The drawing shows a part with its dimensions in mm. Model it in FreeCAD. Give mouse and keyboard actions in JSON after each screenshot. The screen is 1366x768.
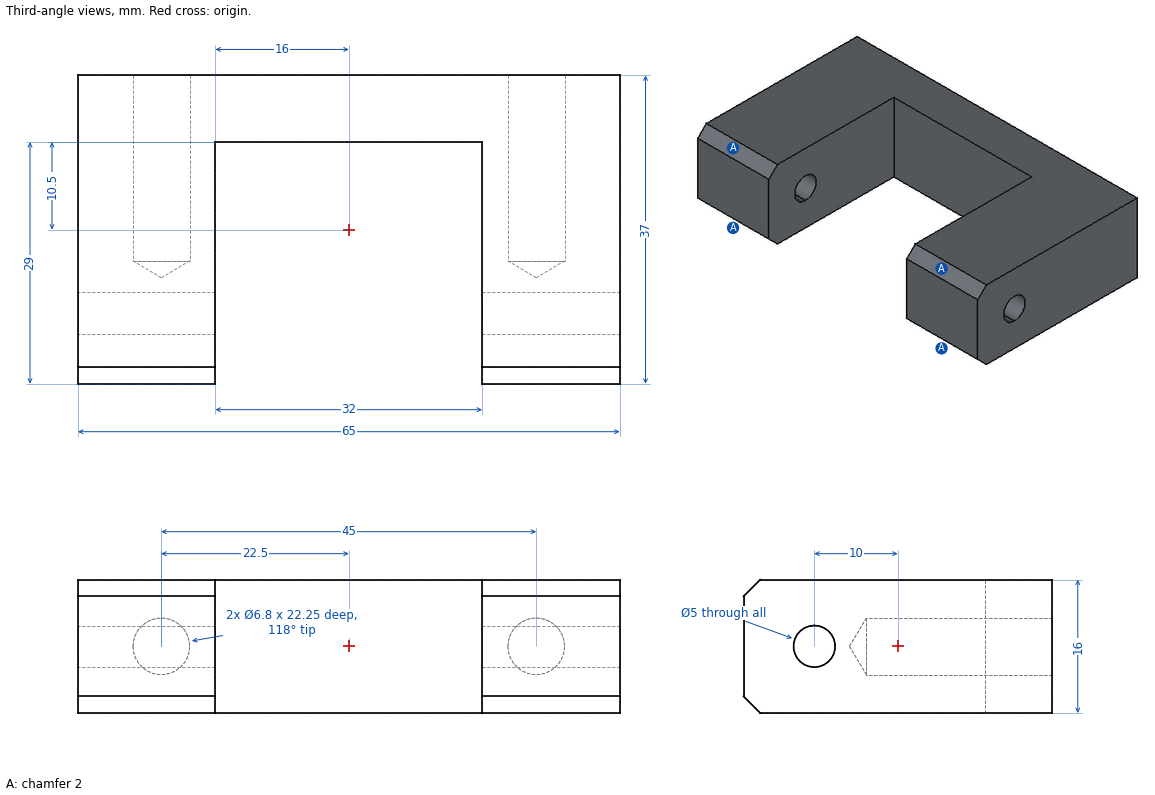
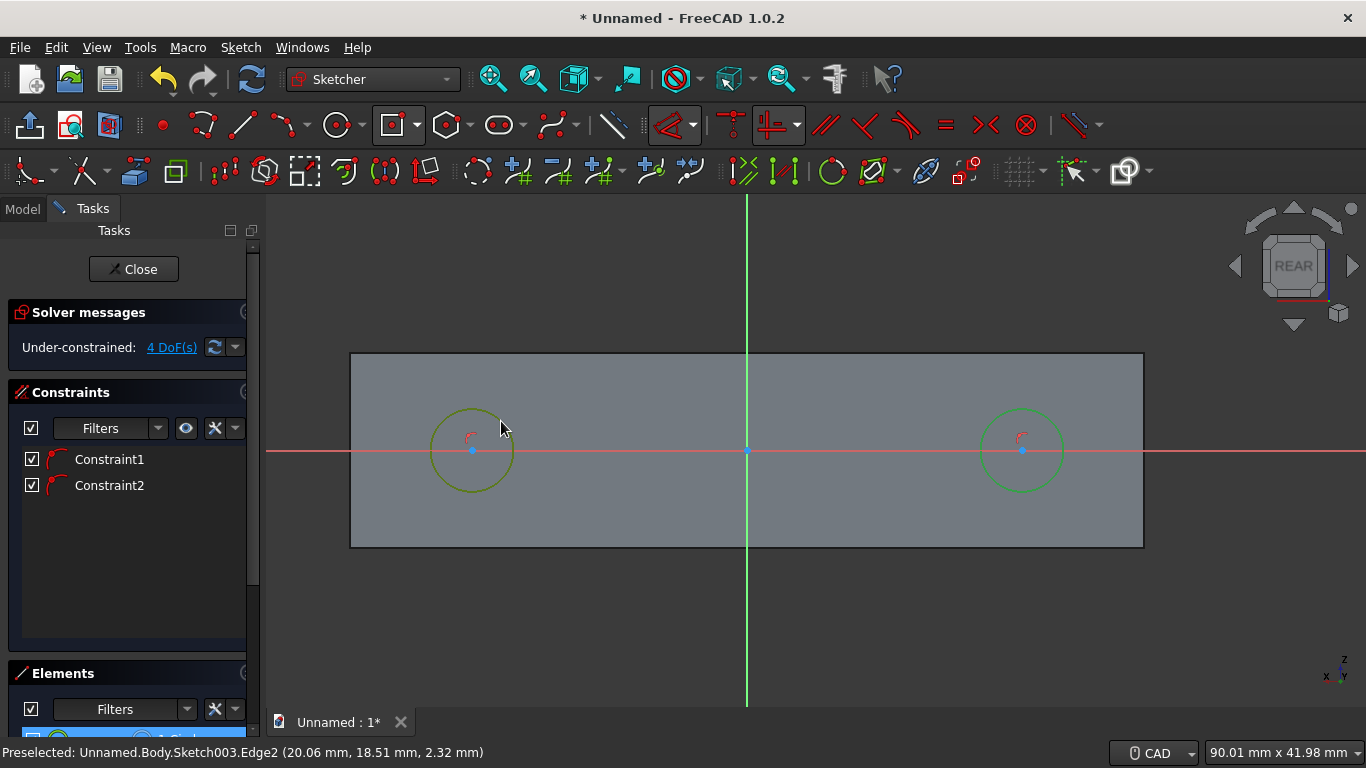
{"action": "left_click", "coordinate": [946, 126]}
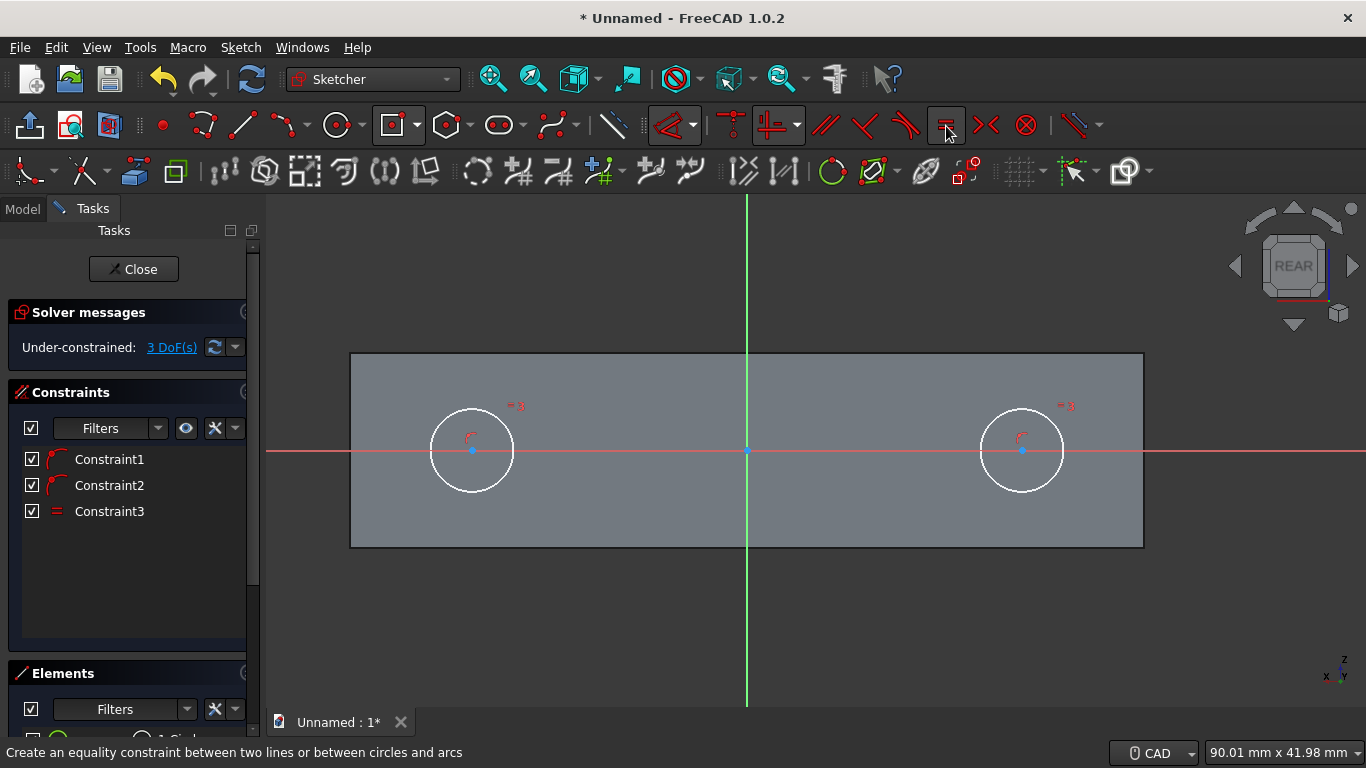
{"action": "left_click", "coordinate": [1051, 421]}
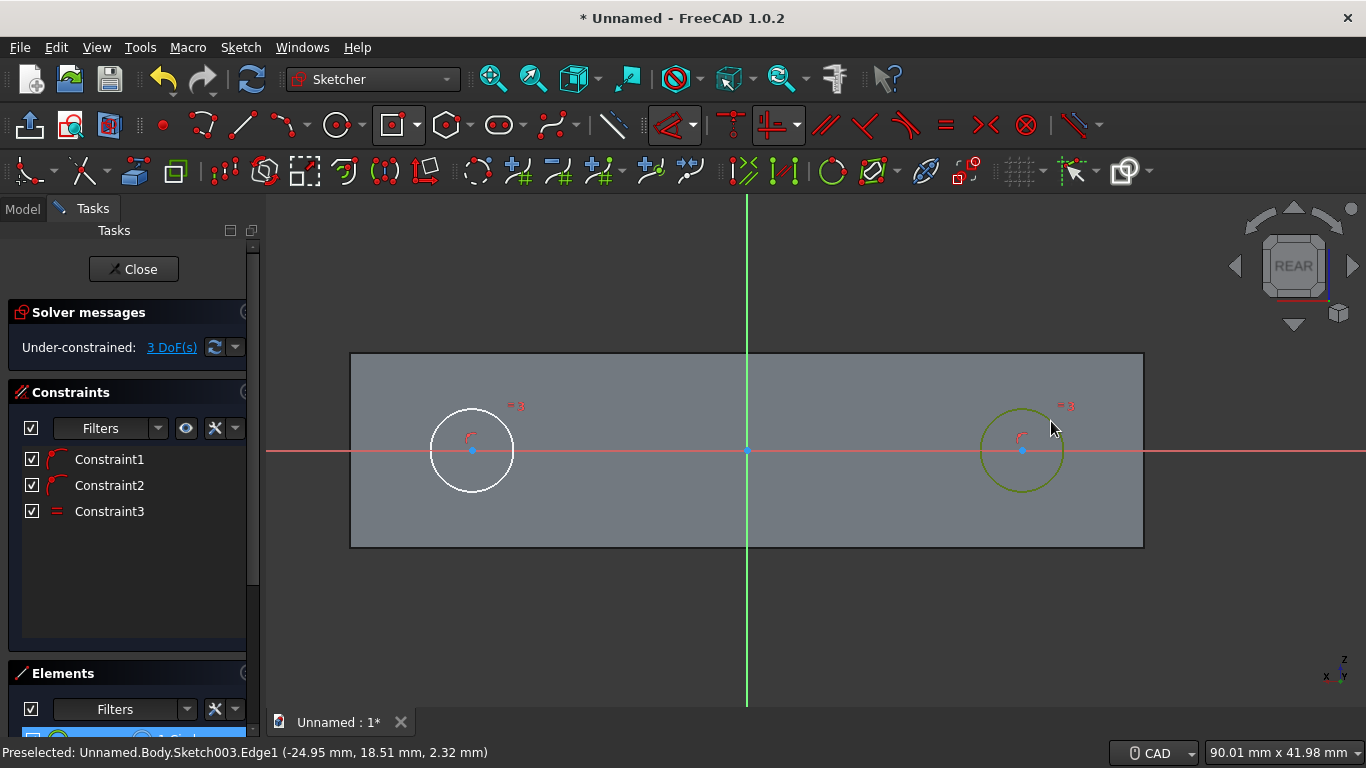
{"action": "left_click", "coordinate": [696, 126]}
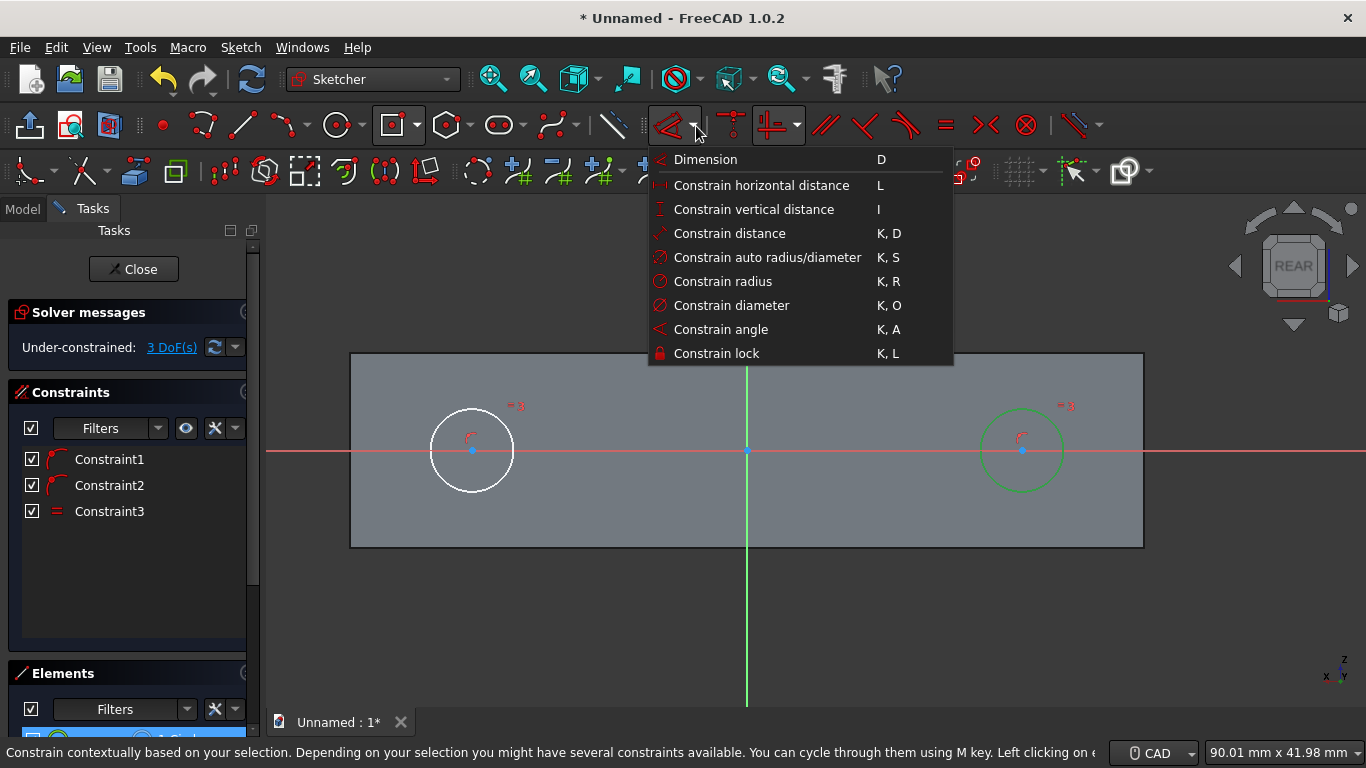
{"action": "left_click", "coordinate": [801, 305]}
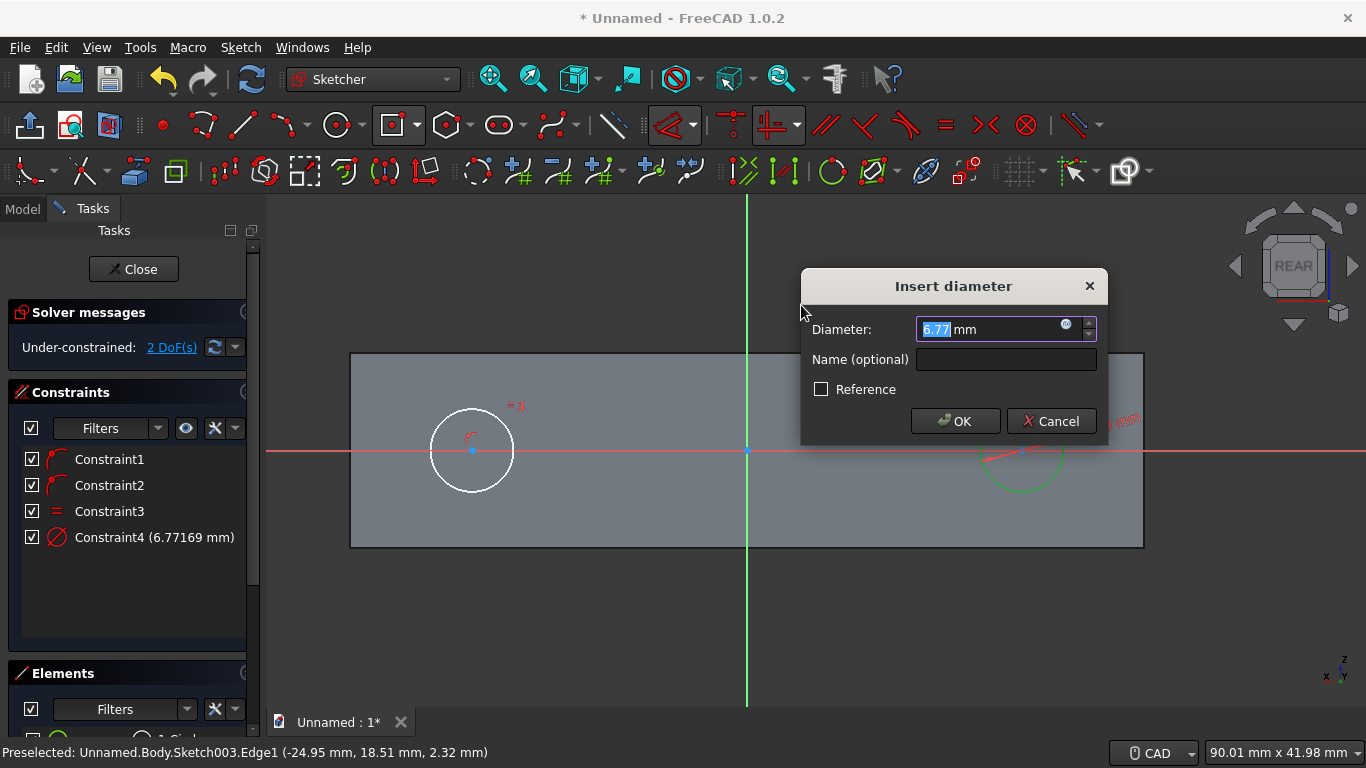
{"action": "type", "text": "6.8"}
{"action": "key", "text": "Return"}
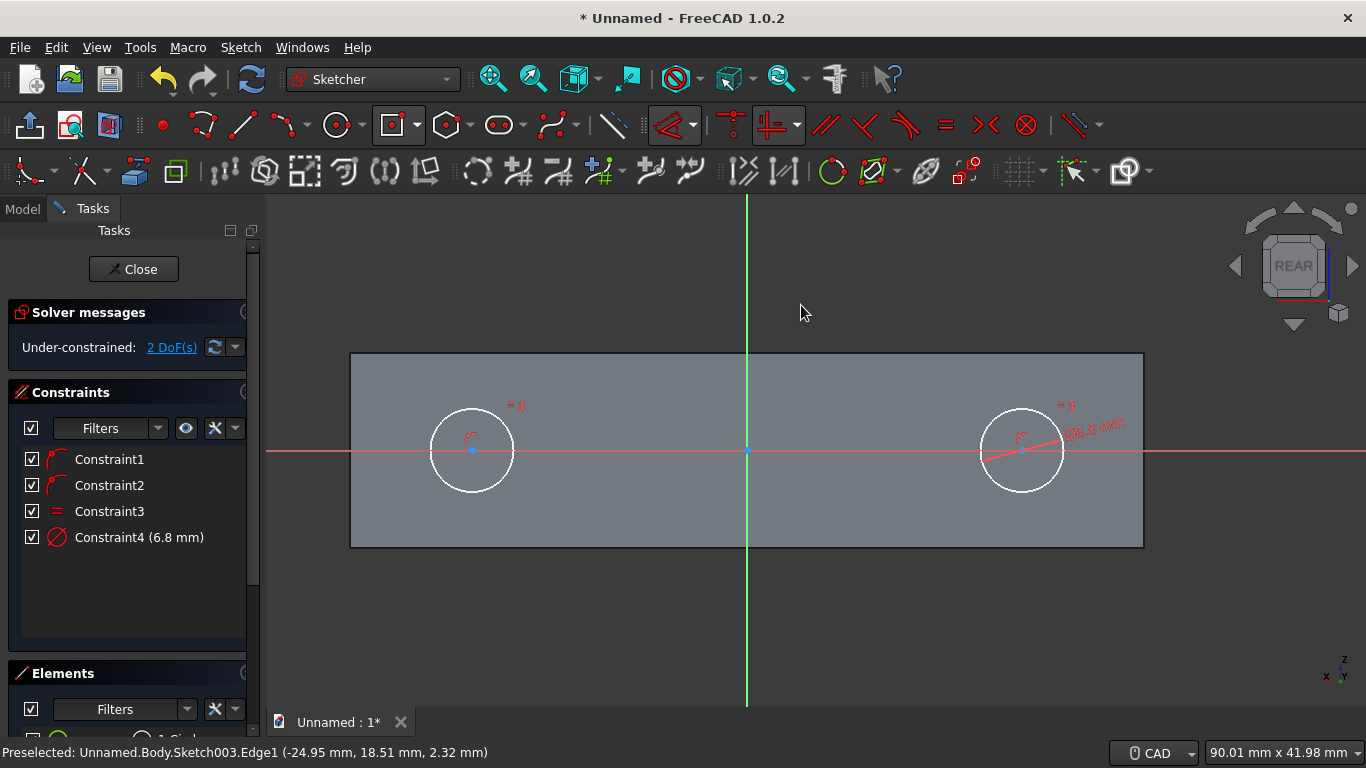
{"action": "left_click", "coordinate": [1022, 450]}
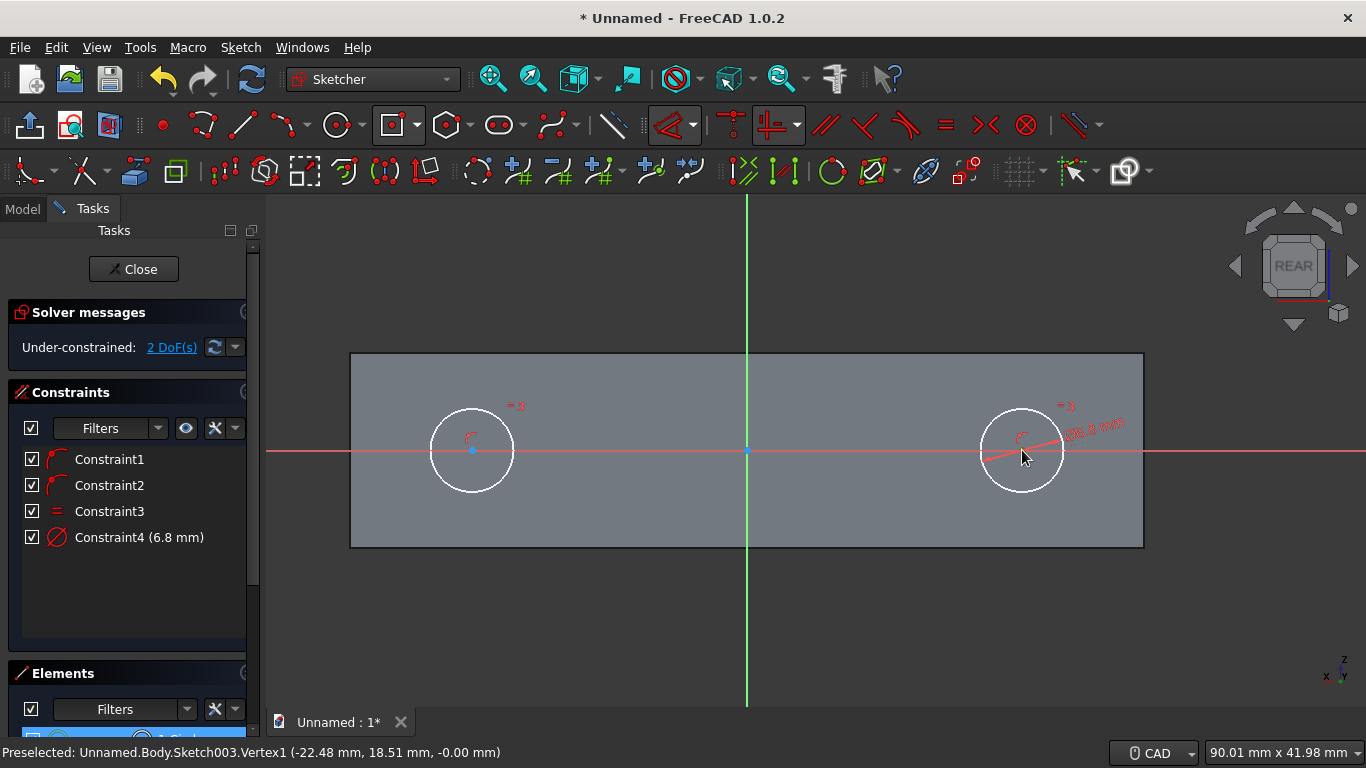
{"action": "left_click", "coordinate": [472, 450]}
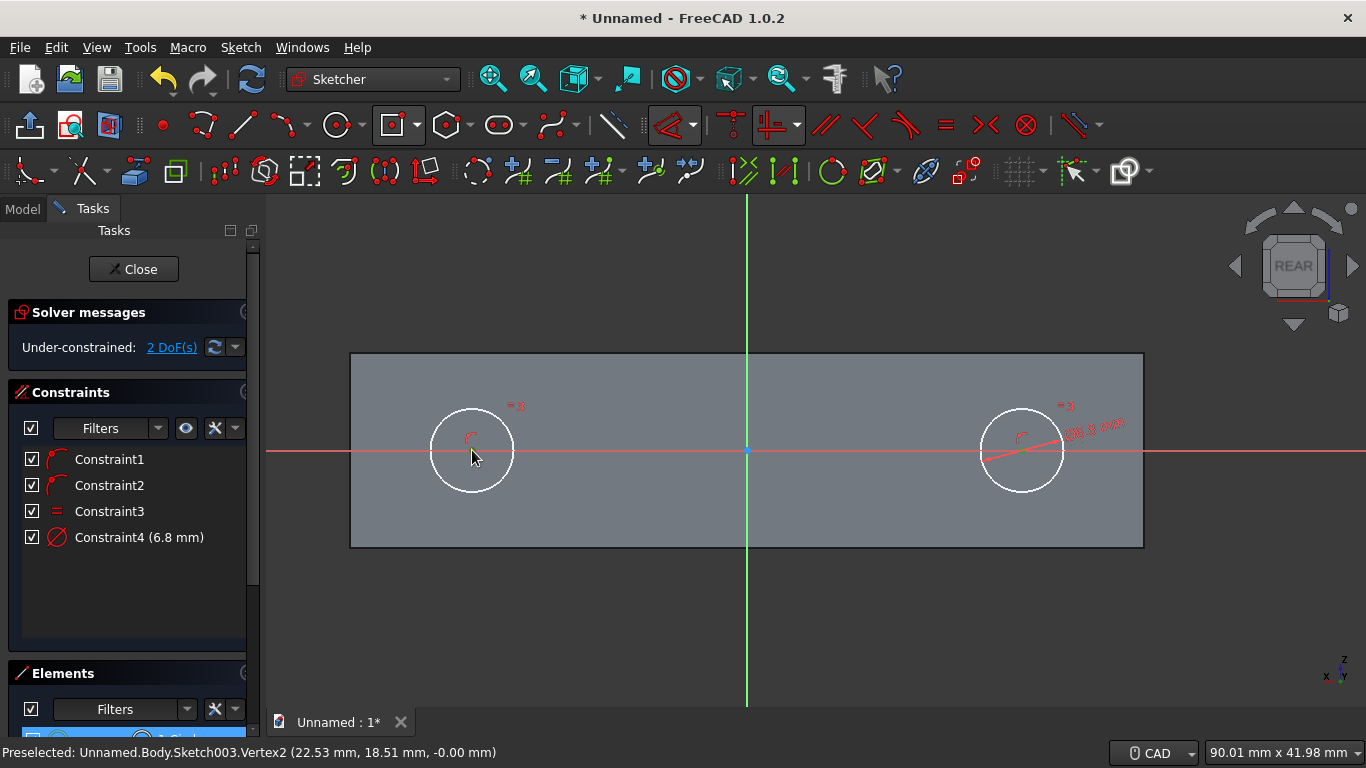
{"action": "key", "text": "l"}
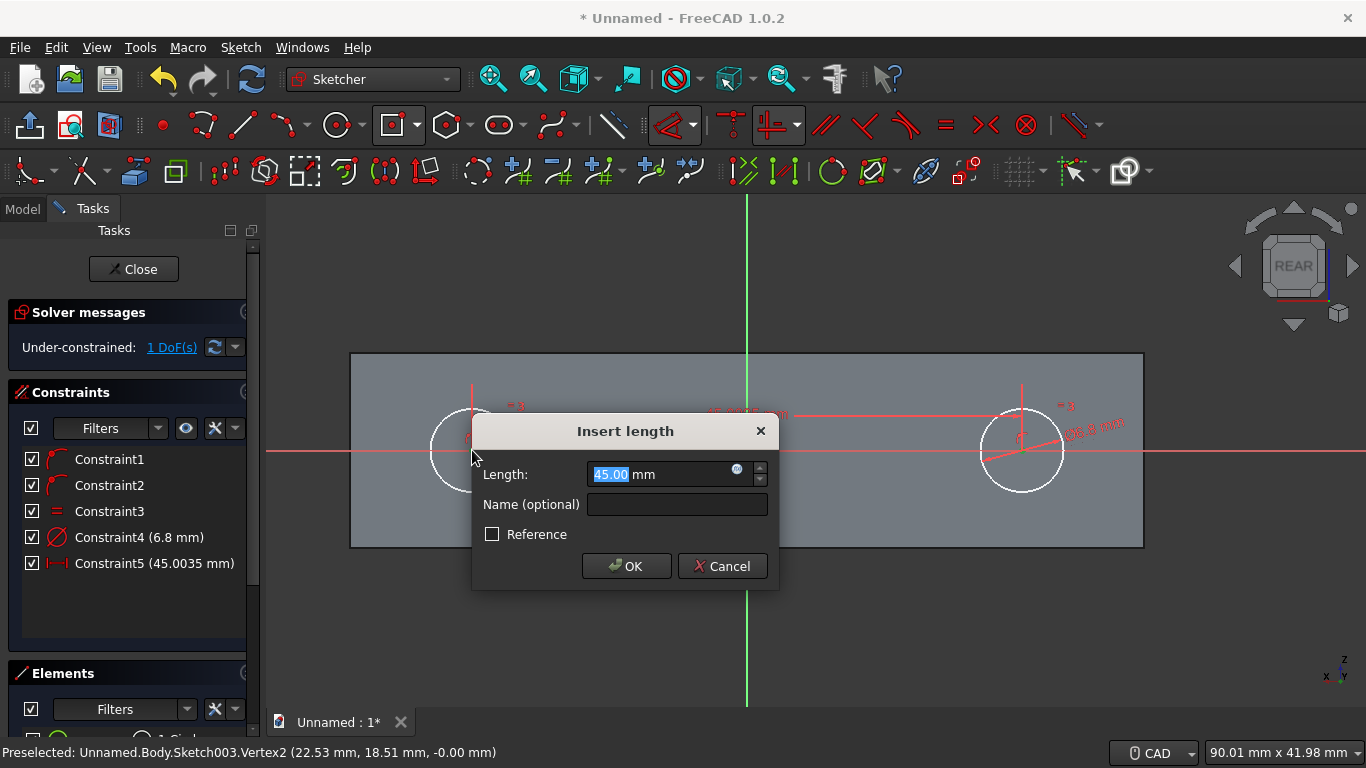
{"action": "type", "text": "45"}
{"action": "key", "text": "Return"}